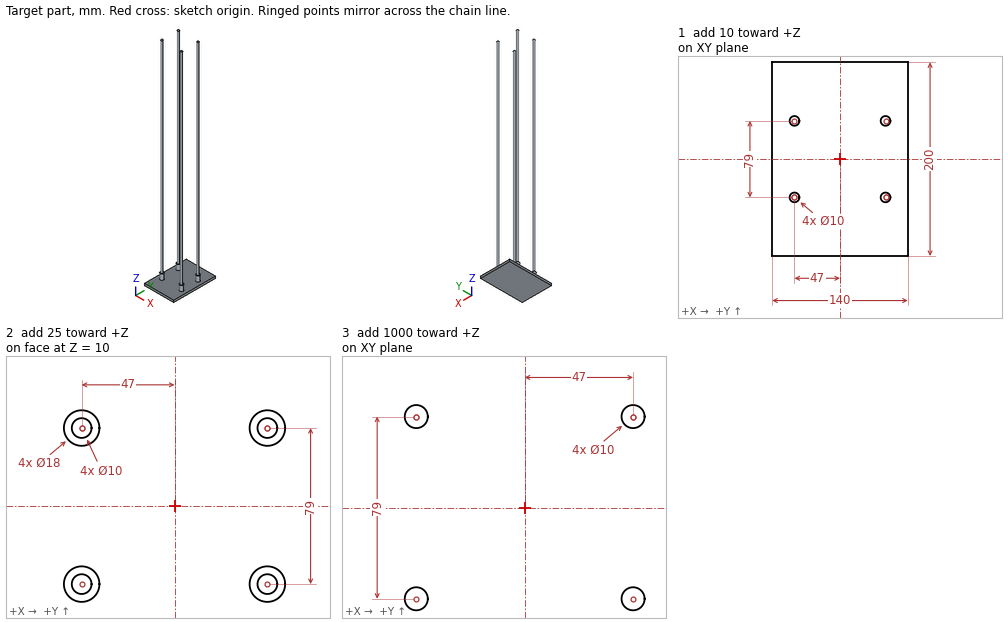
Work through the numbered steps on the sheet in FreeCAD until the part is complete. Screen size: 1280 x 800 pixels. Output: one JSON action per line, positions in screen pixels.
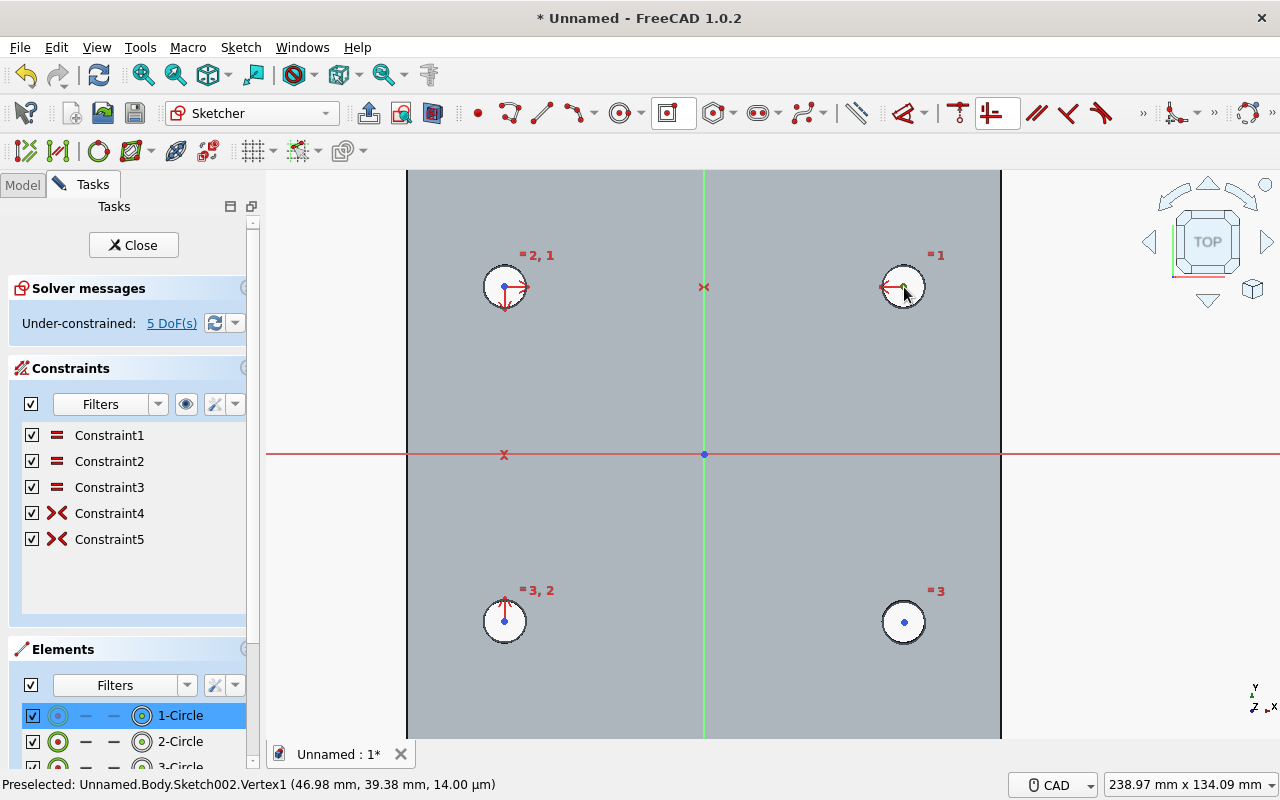
{"action": "left_click", "coordinate": [904, 623]}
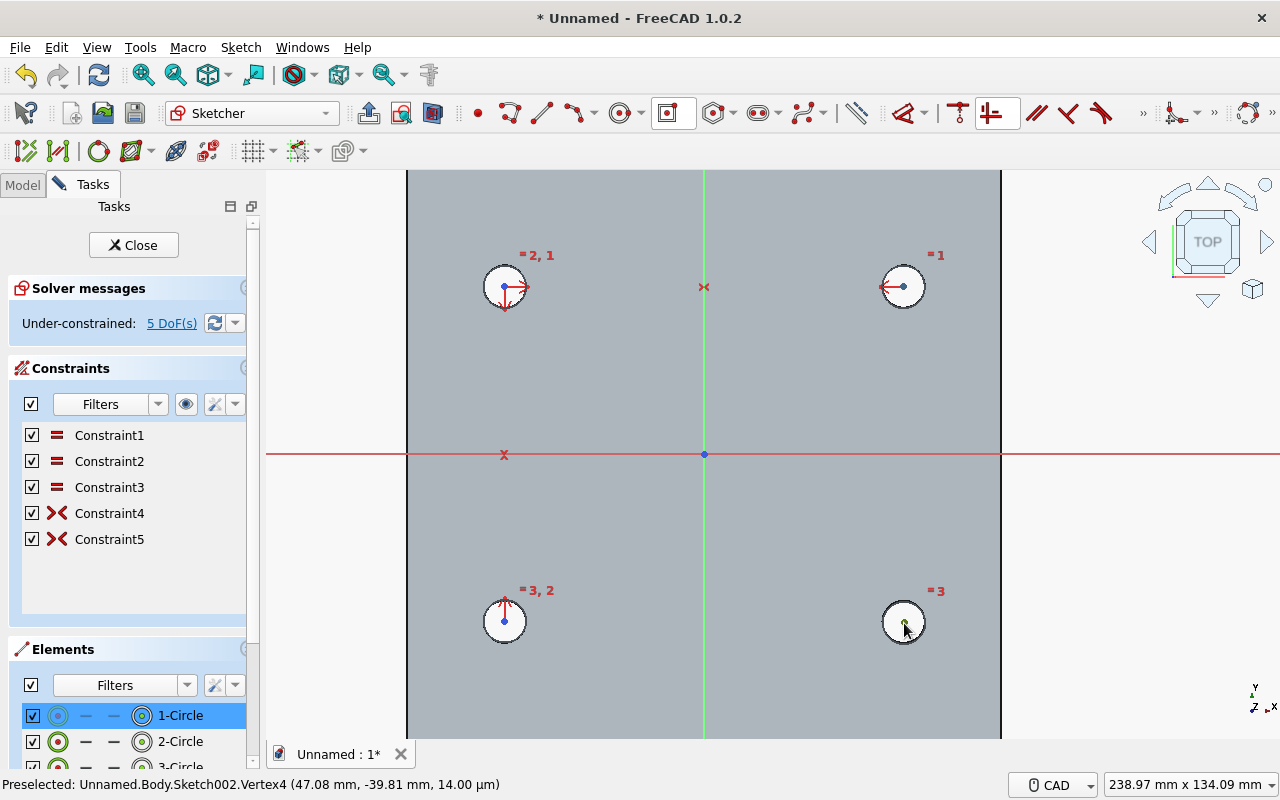
{"action": "left_click", "coordinate": [353, 454]}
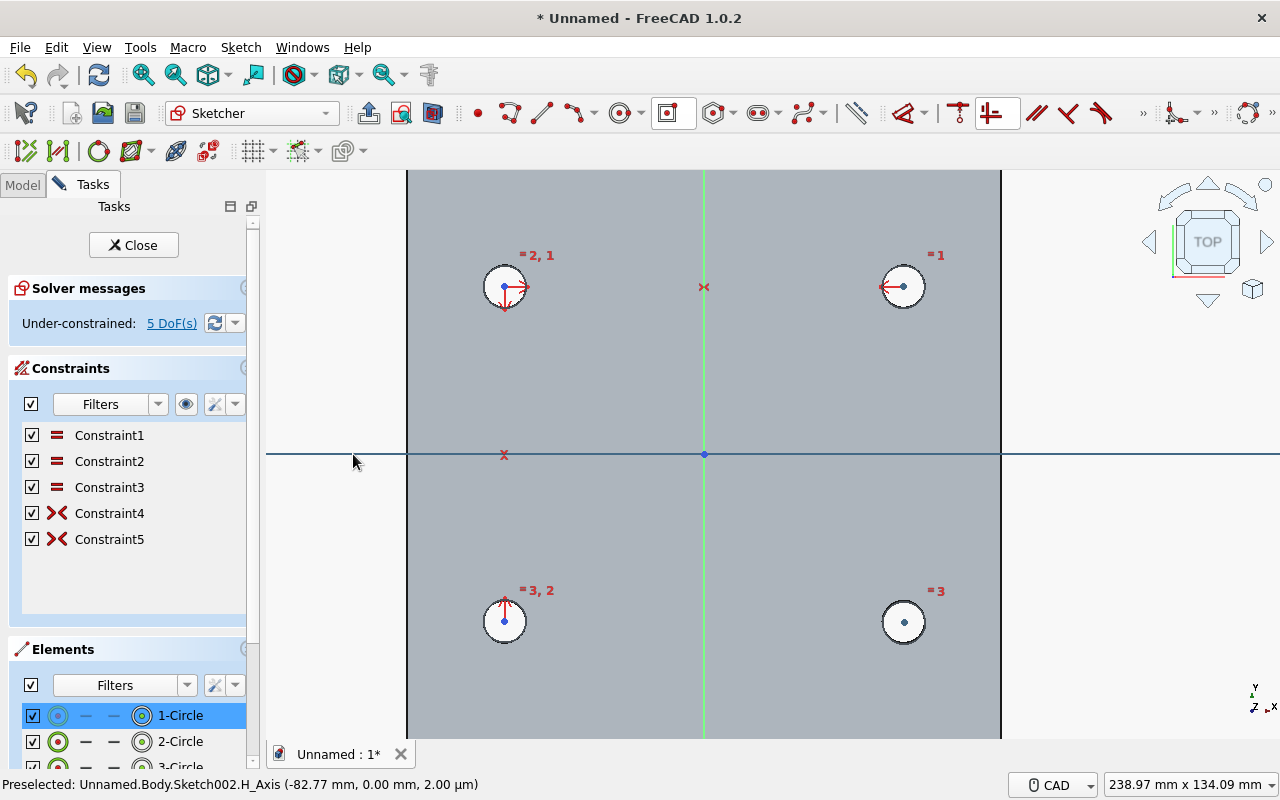
{"action": "key", "text": "s"}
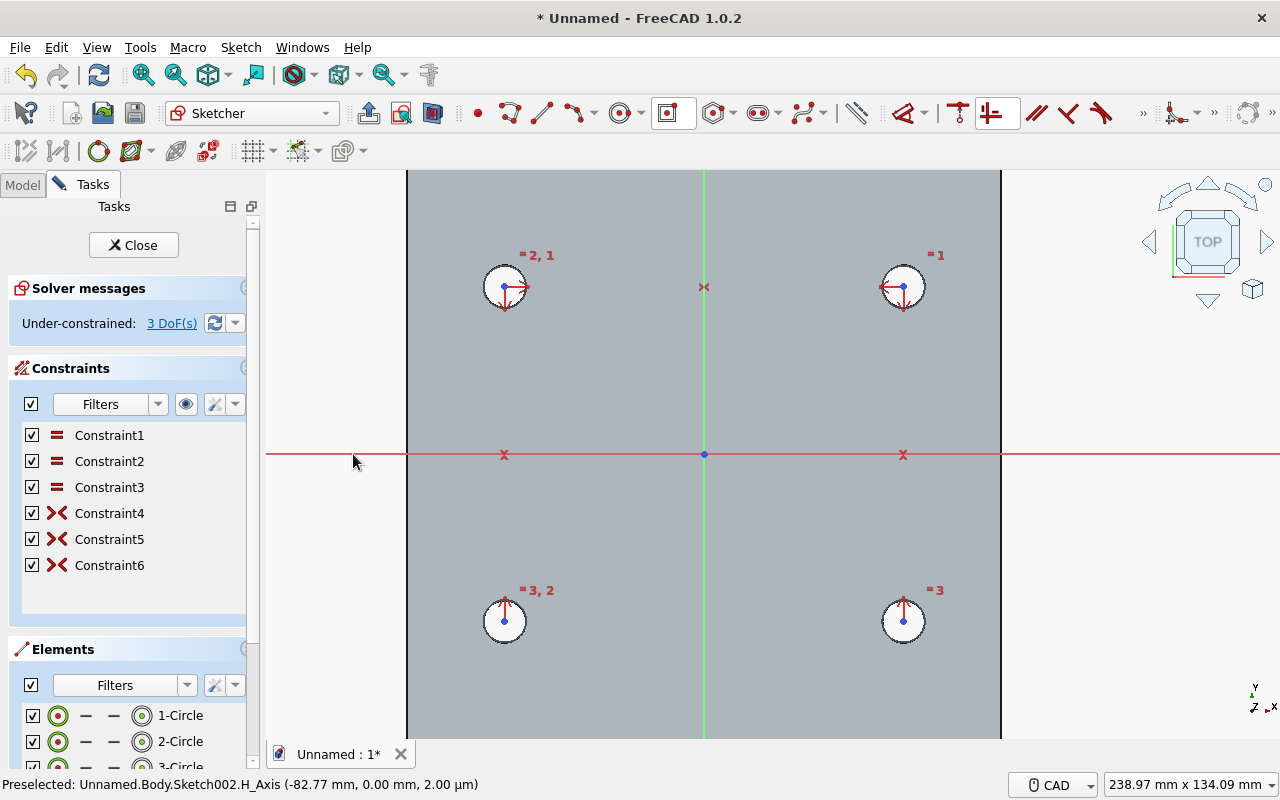
{"action": "left_click", "coordinate": [904, 114]}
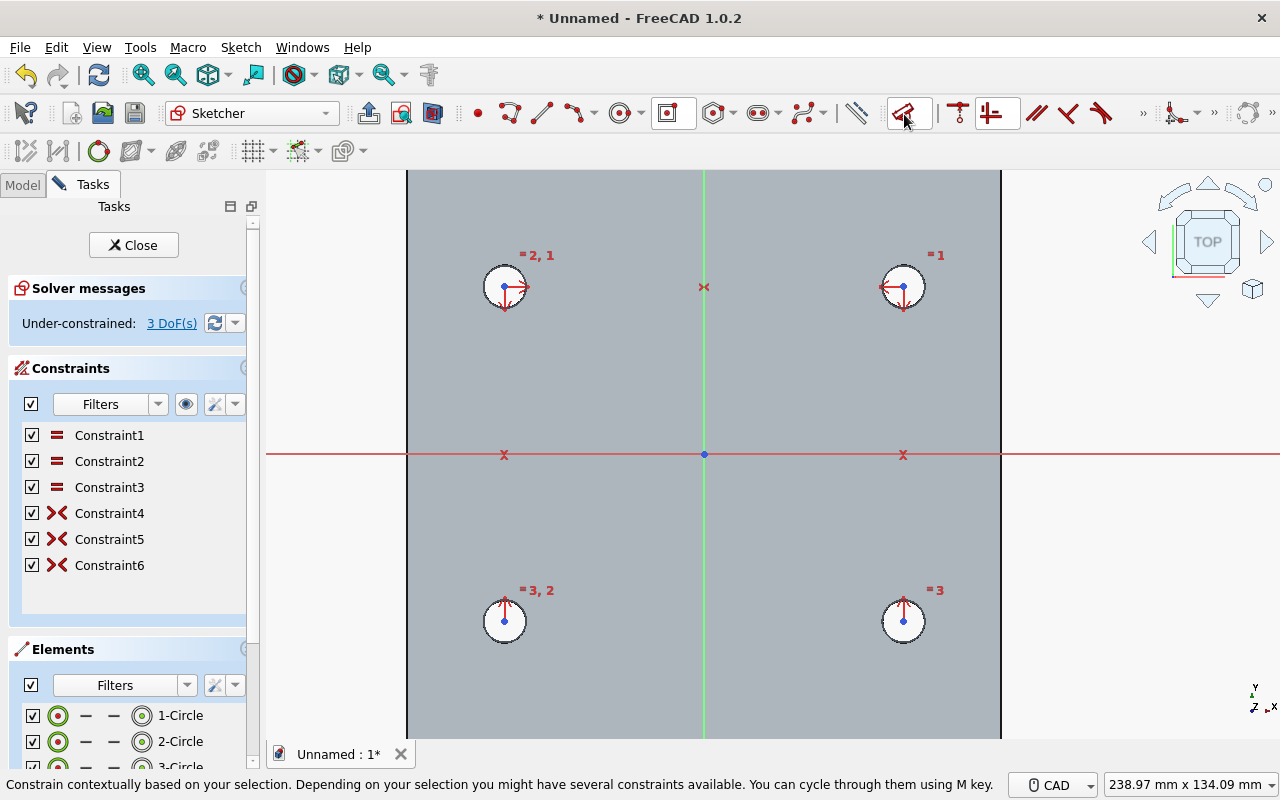
{"action": "left_click", "coordinate": [919, 272]}
{"action": "left_click", "coordinate": [942, 250]}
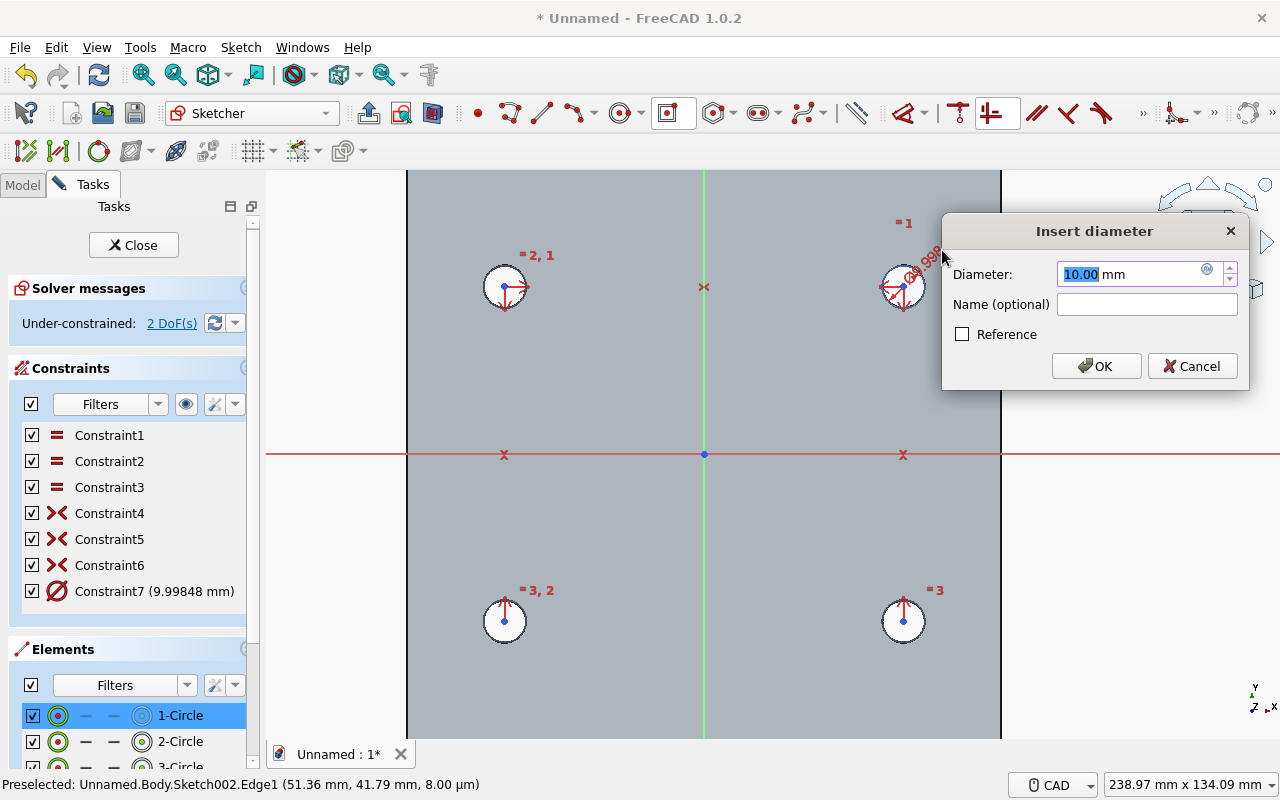
{"action": "type", "text": "10"}
{"action": "key", "text": "Return"}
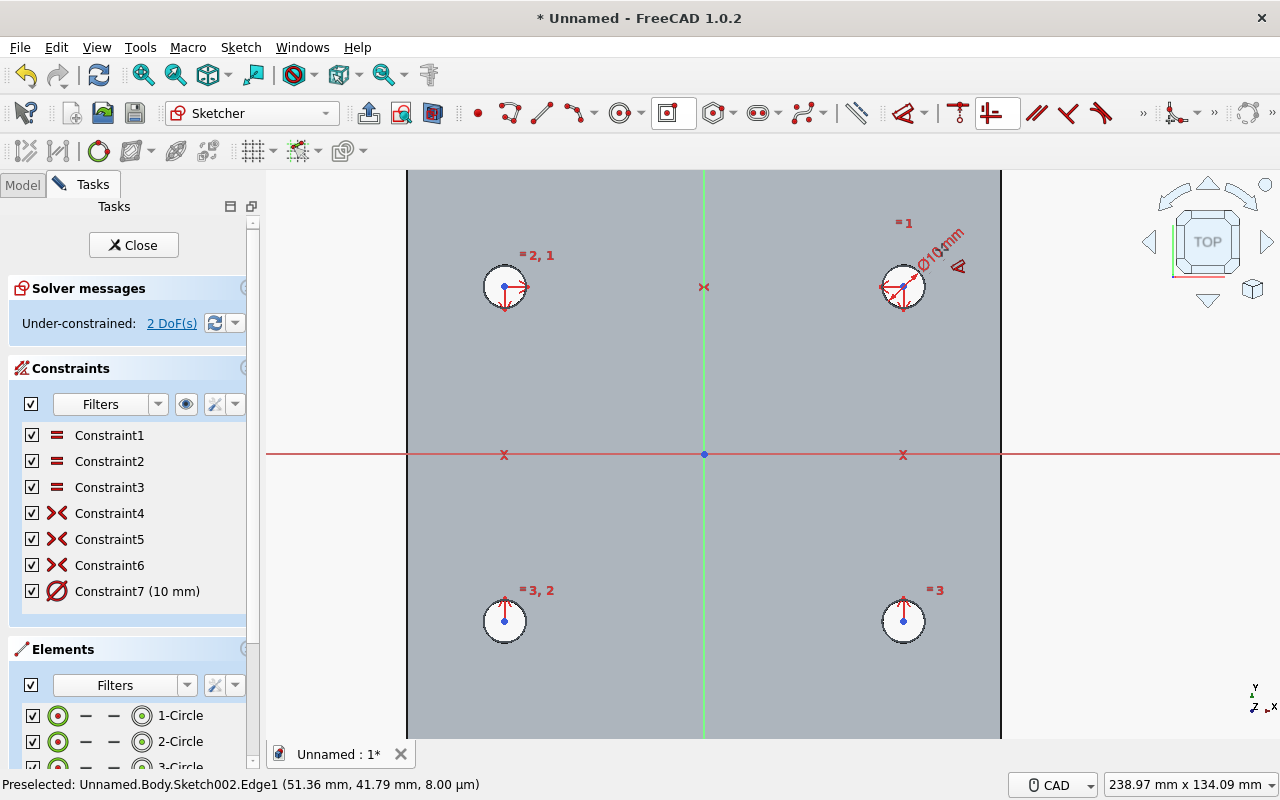
{"action": "left_click", "coordinate": [904, 287]}
{"action": "left_click", "coordinate": [804, 253]}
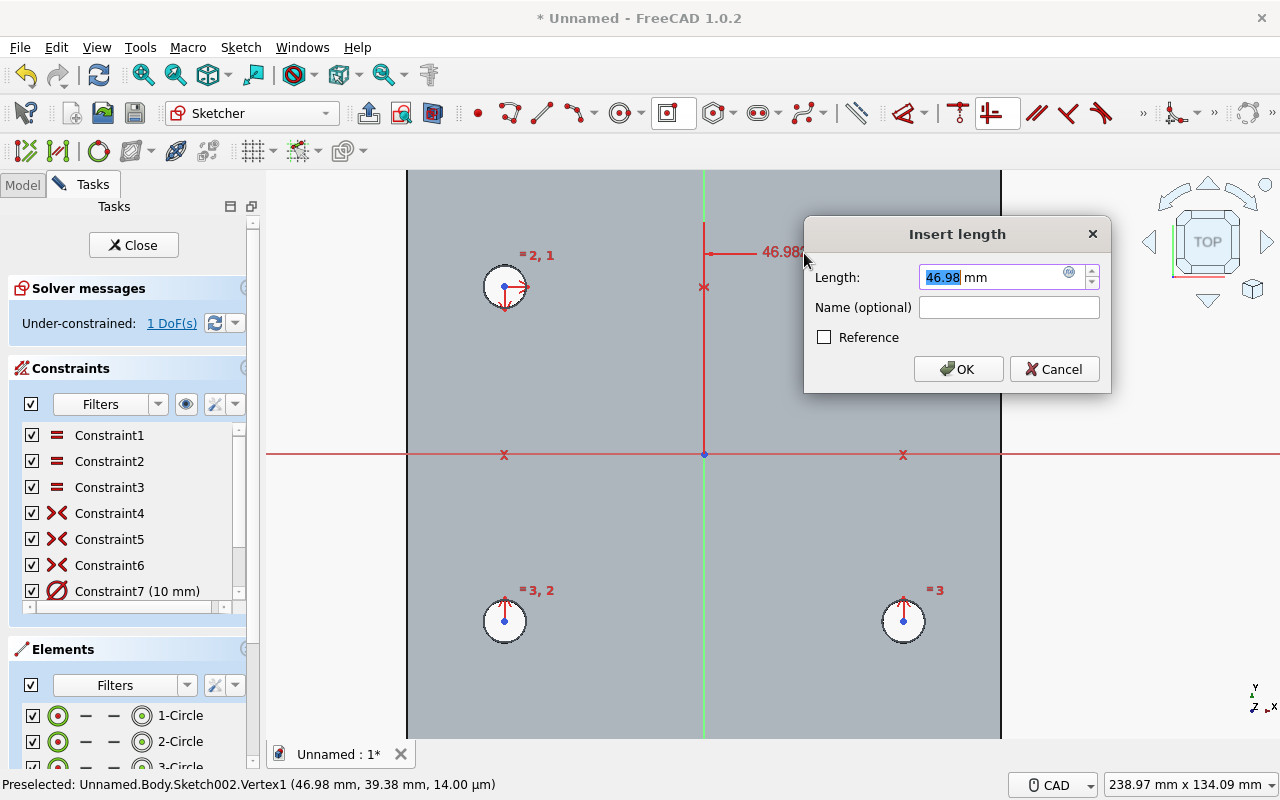
{"action": "type", "text": "47"}
{"action": "key", "text": "Return"}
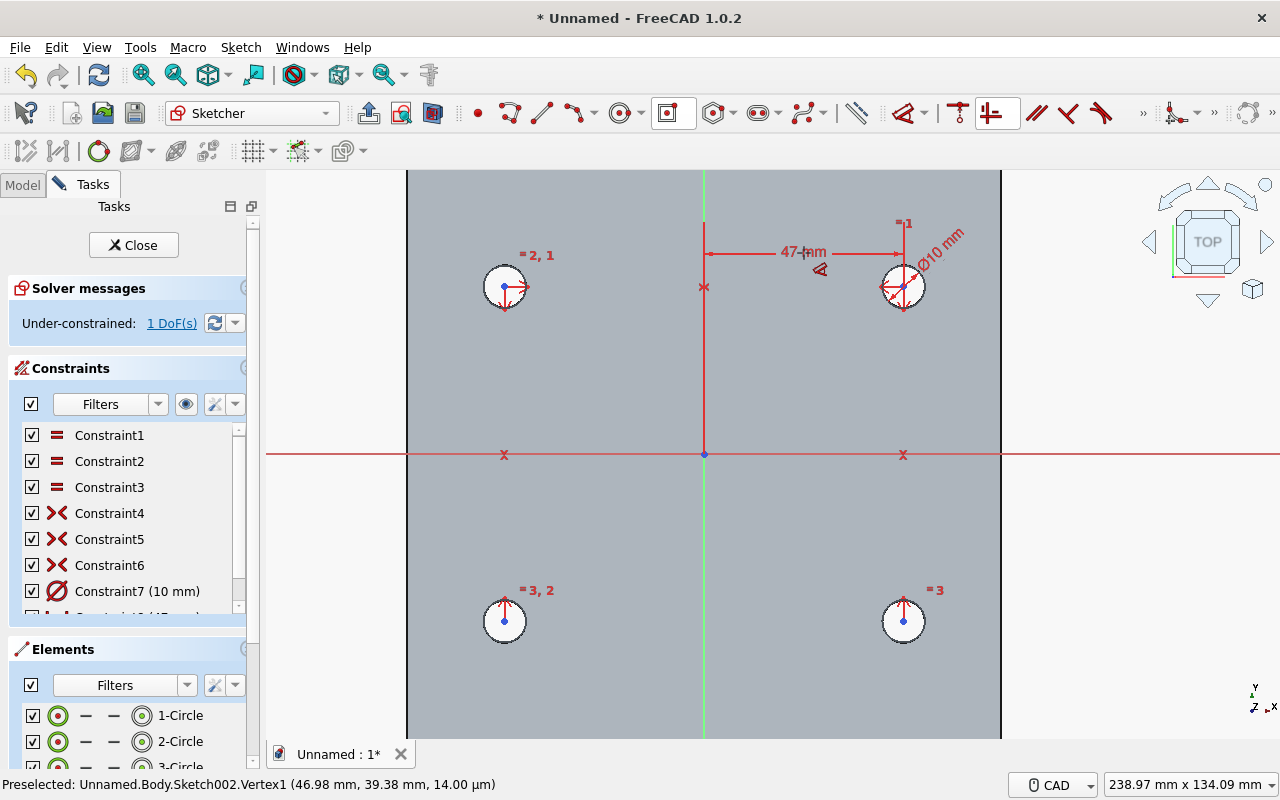
{"action": "left_click", "coordinate": [505, 287]}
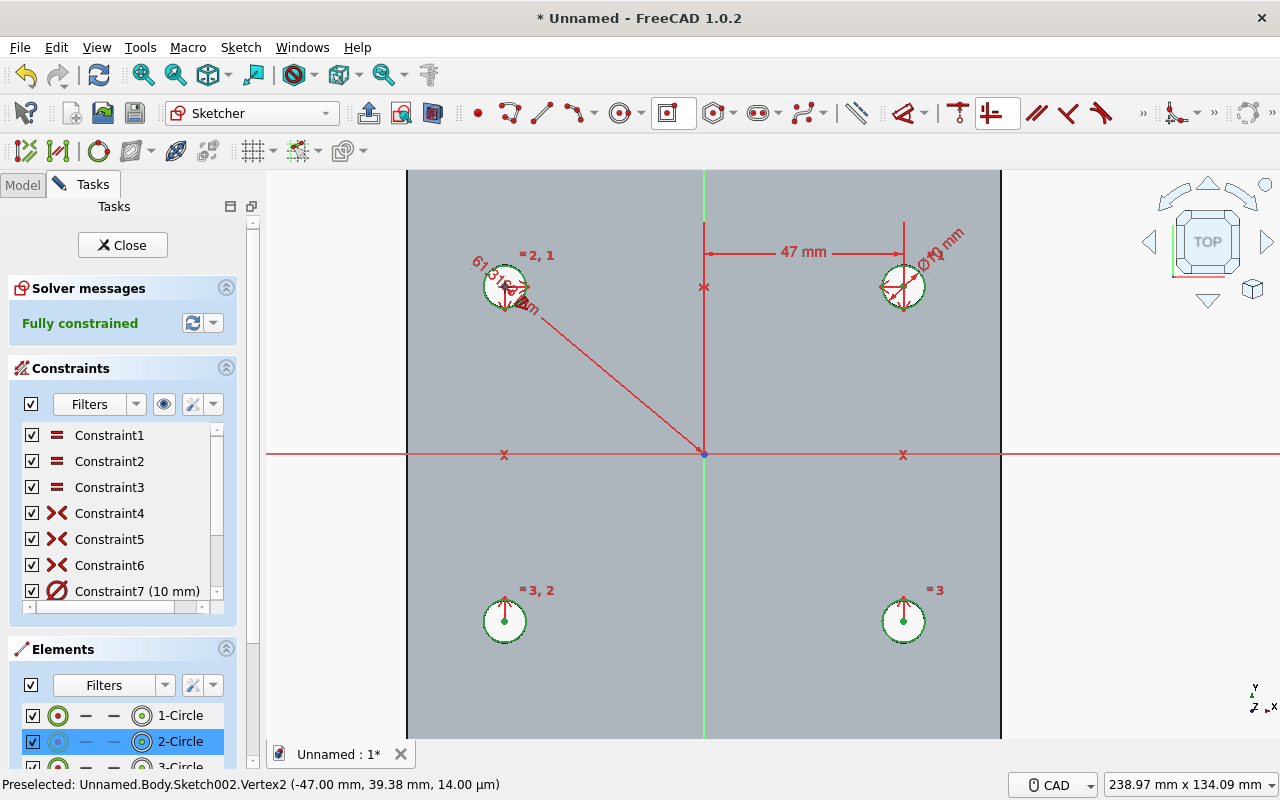
{"action": "left_click", "coordinate": [505, 621]}
{"action": "left_click", "coordinate": [471, 377]}